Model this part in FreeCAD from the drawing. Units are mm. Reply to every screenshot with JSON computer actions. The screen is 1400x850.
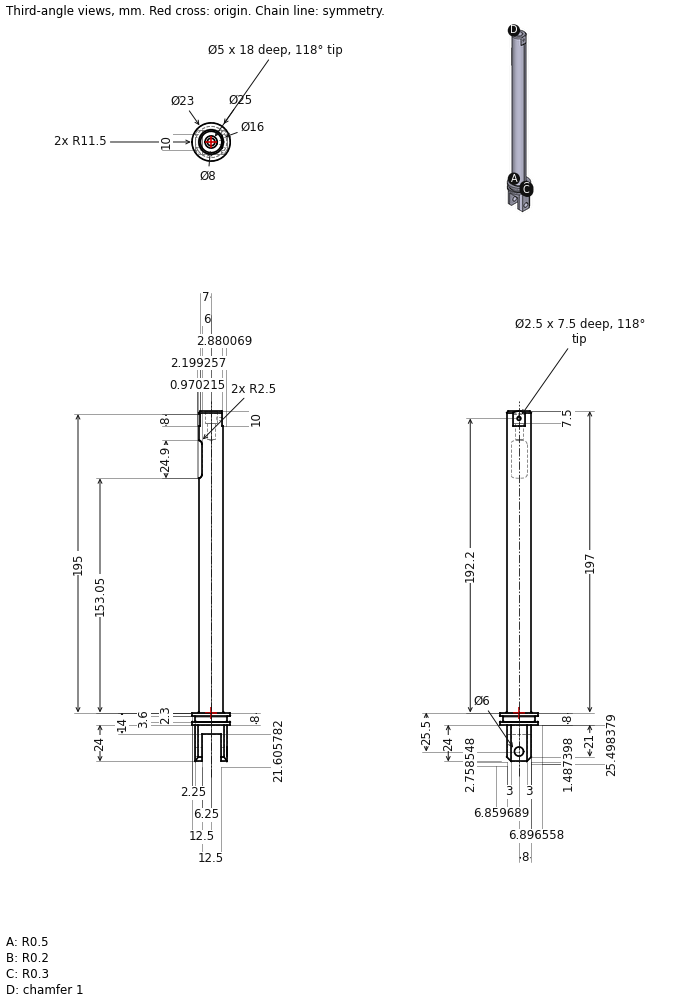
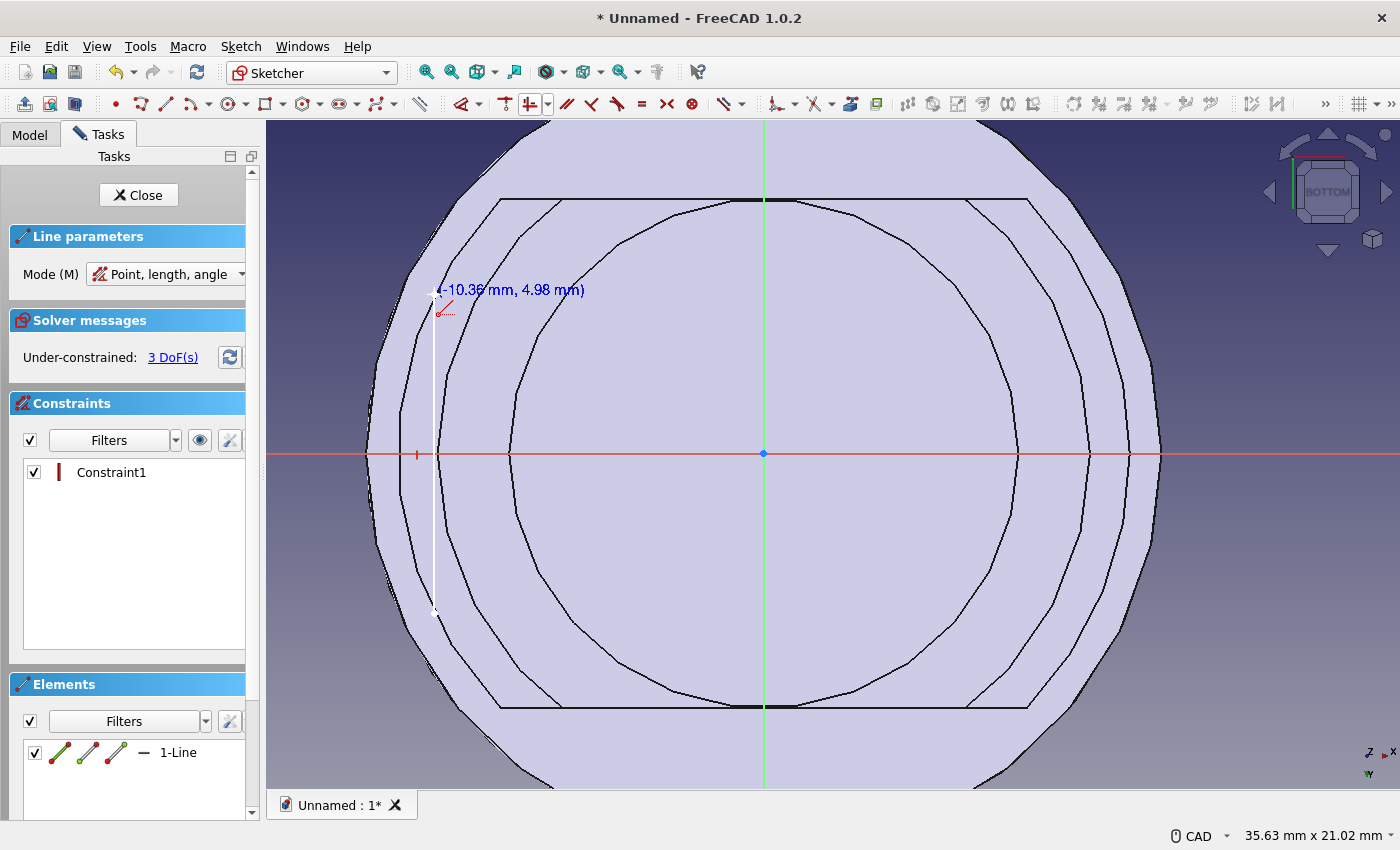
{"action": "left_click", "coordinate": [208, 104]}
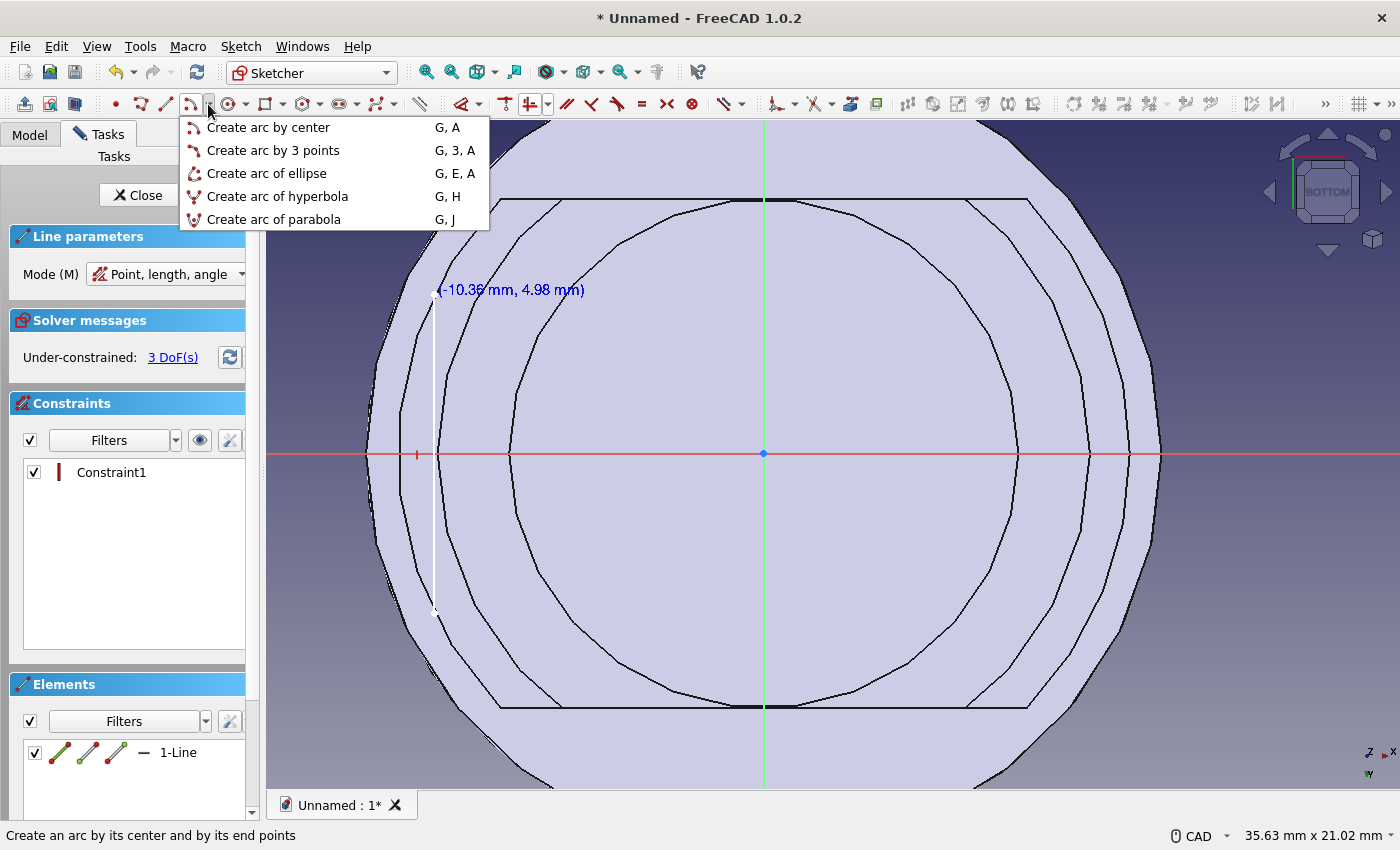
{"action": "left_click", "coordinate": [334, 150]}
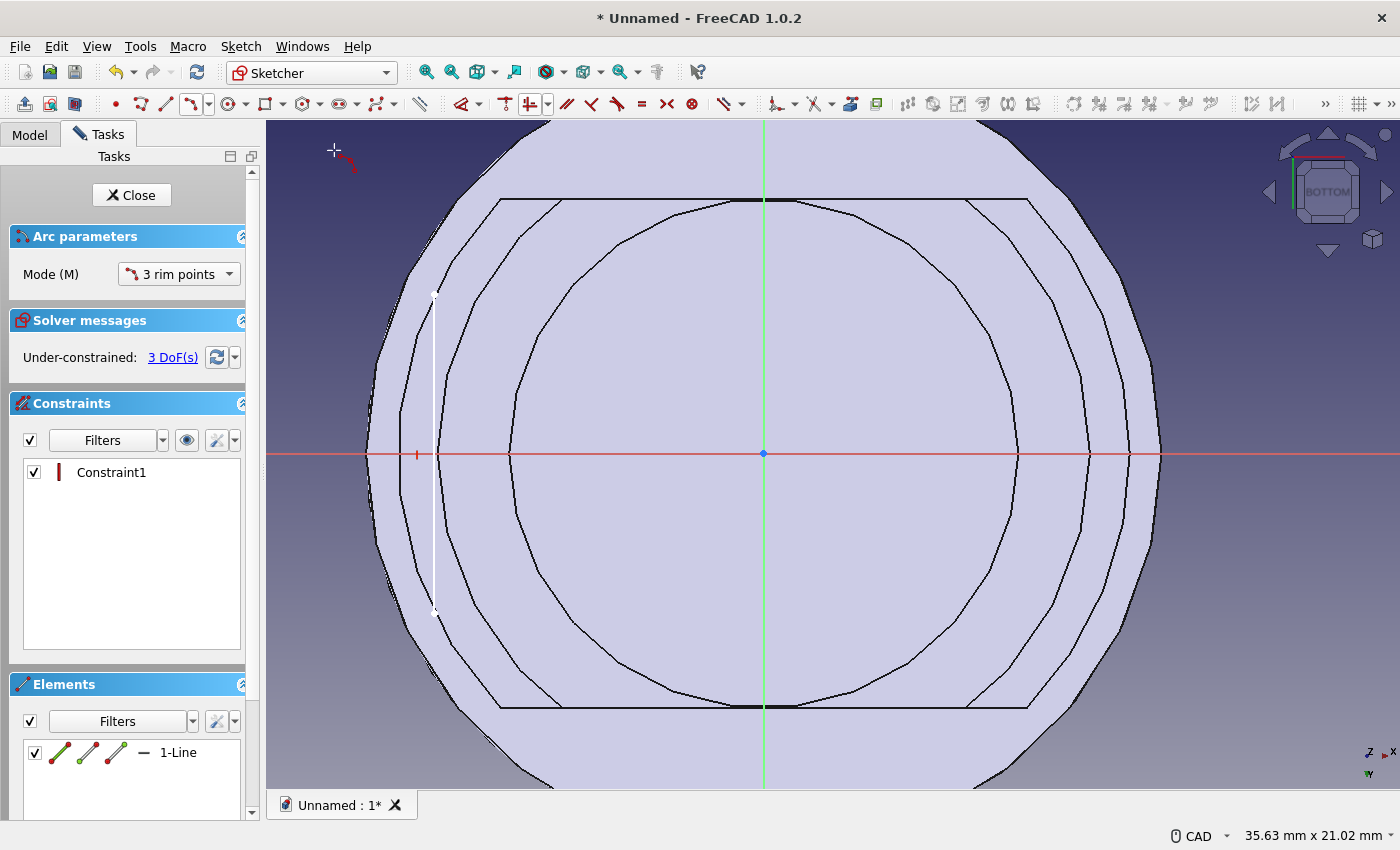
{"action": "left_click", "coordinate": [434, 295]}
{"action": "left_click", "coordinate": [434, 614]}
{"action": "left_click", "coordinate": [399, 421]}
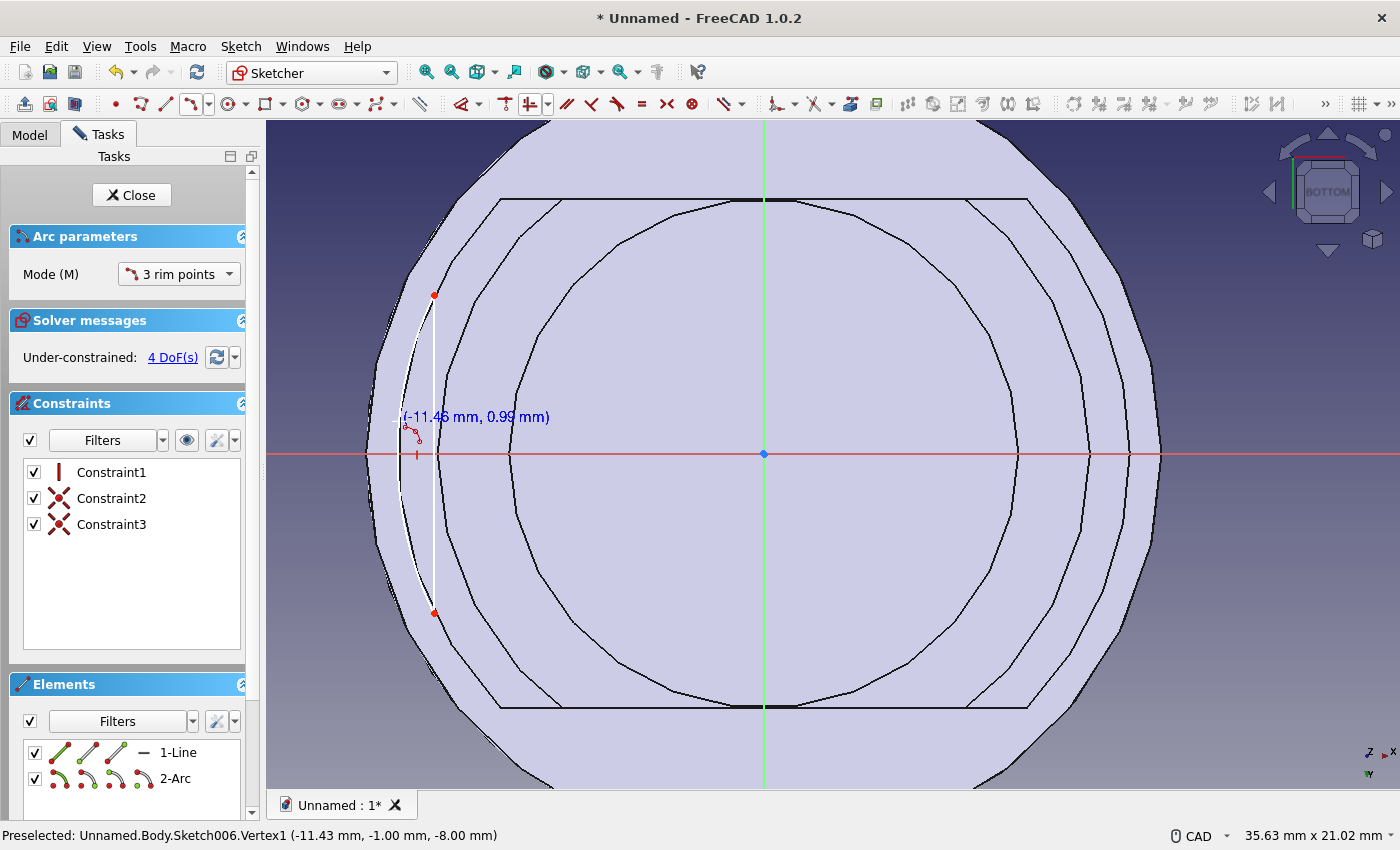
{"action": "left_click", "coordinate": [166, 104]}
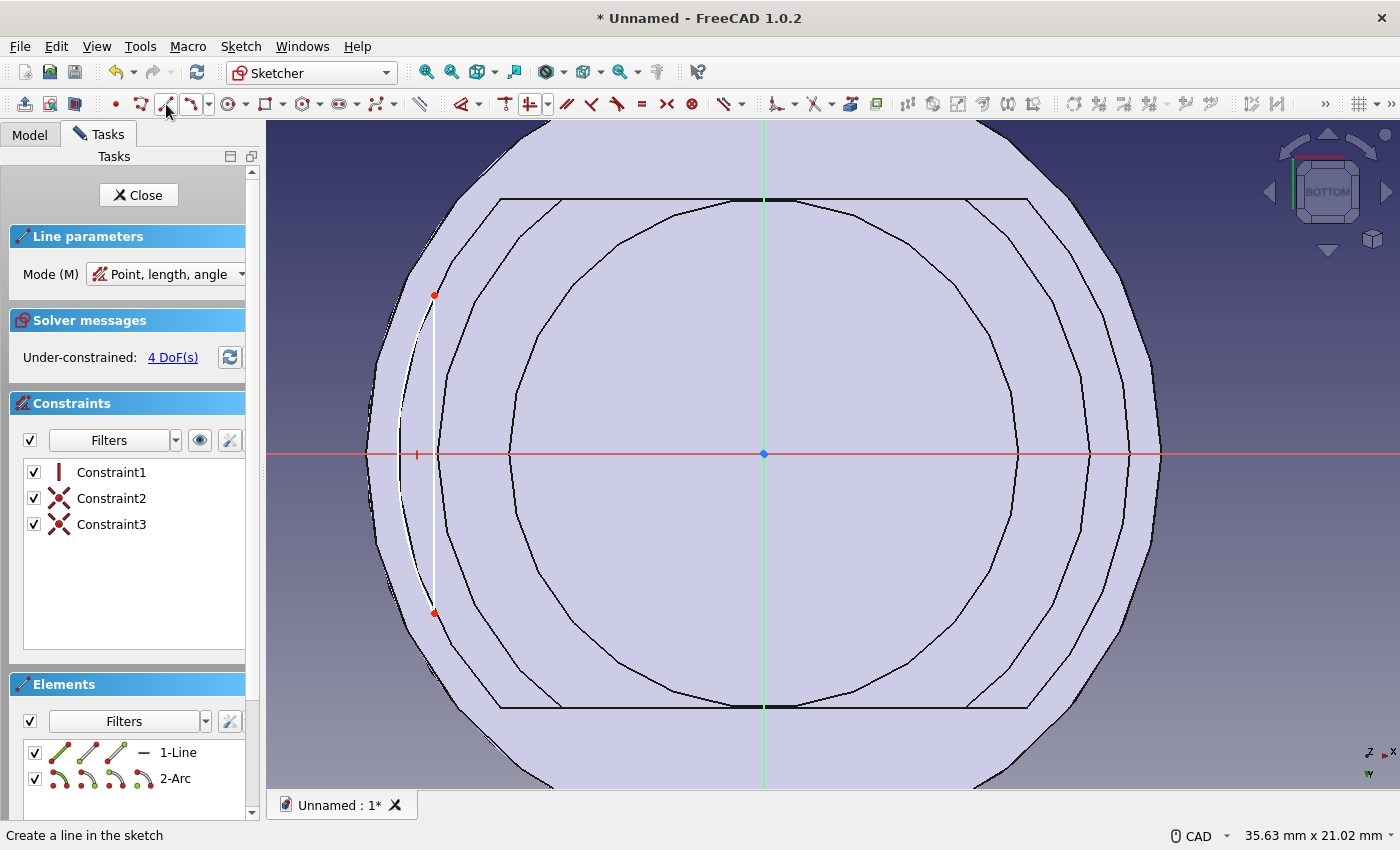
{"action": "left_click", "coordinate": [1093, 294]}
{"action": "left_click", "coordinate": [1093, 613]}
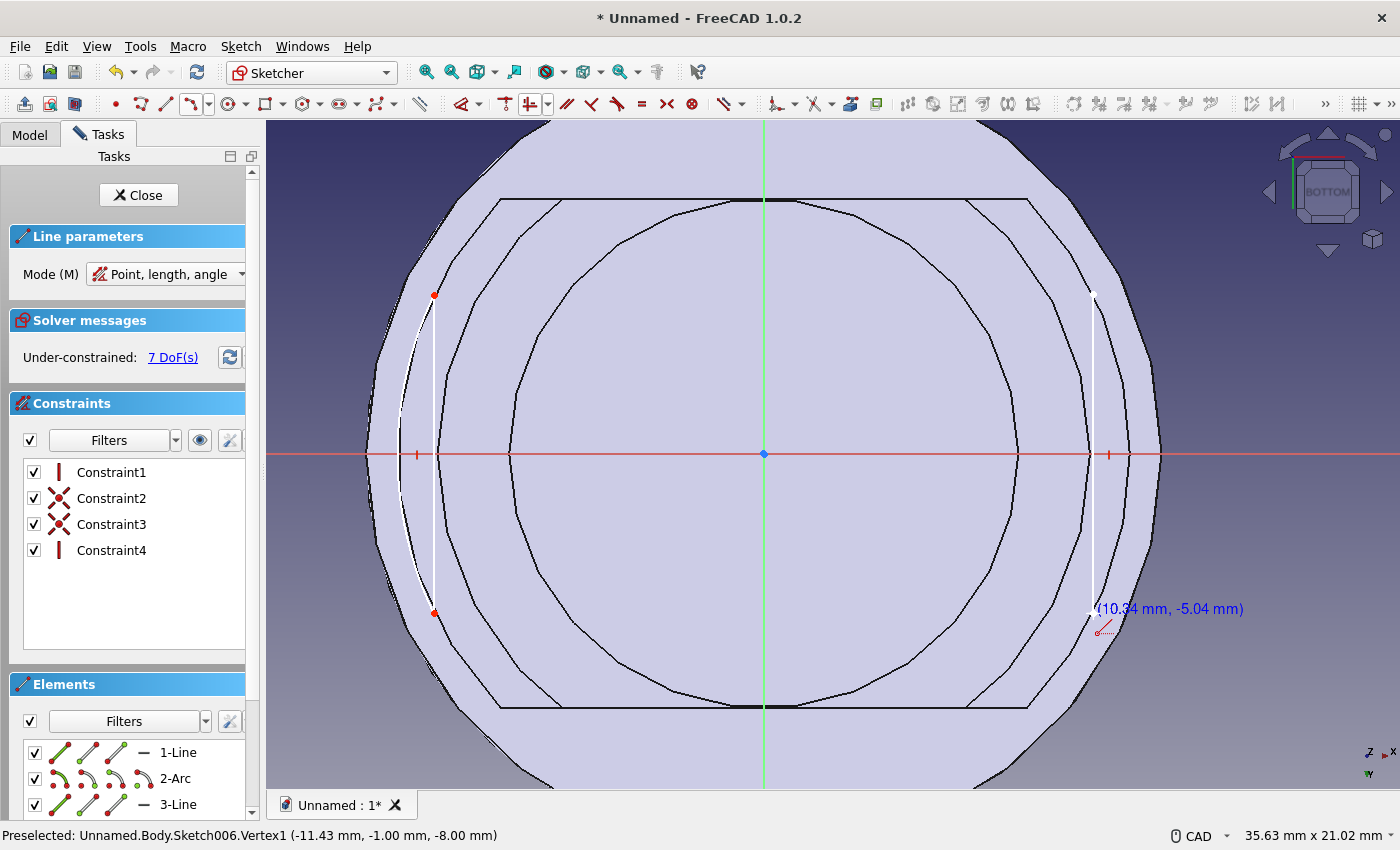
{"action": "left_click", "coordinate": [190, 104]}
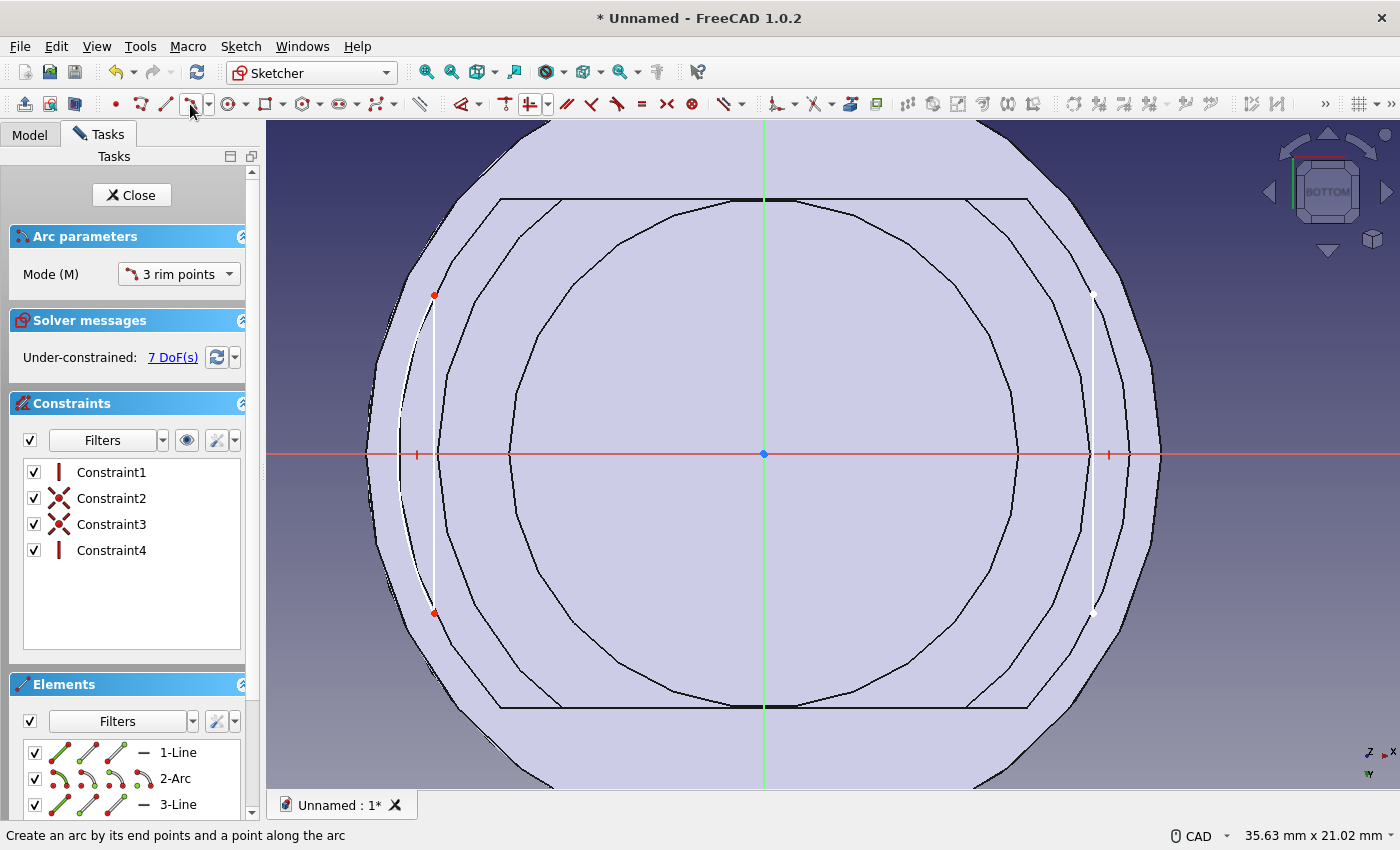
{"action": "left_click", "coordinate": [1093, 614]}
{"action": "left_click", "coordinate": [1093, 295]}
{"action": "left_click", "coordinate": [1128, 486]}
{"action": "key", "text": "Escape"}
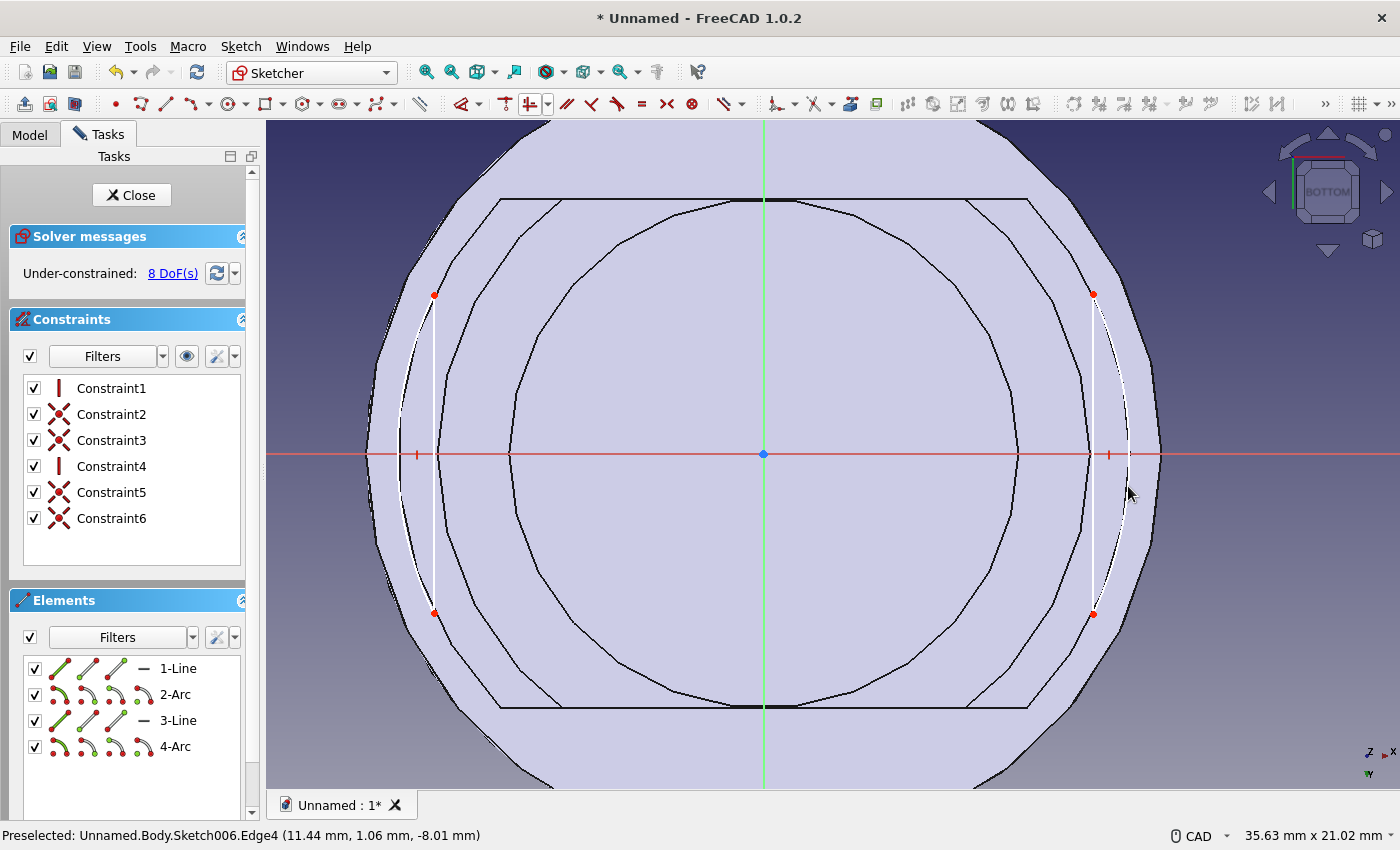
{"action": "left_click", "coordinate": [403, 389]}